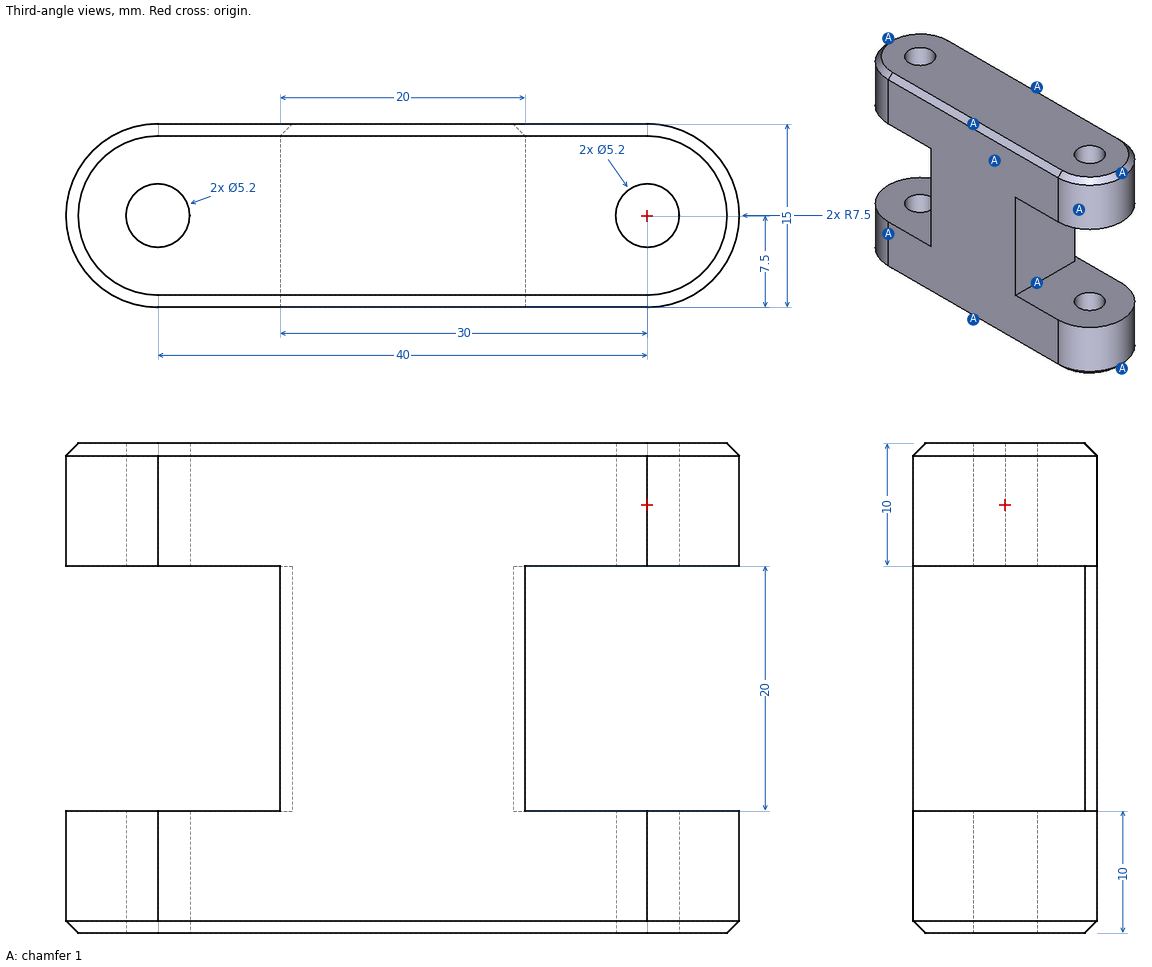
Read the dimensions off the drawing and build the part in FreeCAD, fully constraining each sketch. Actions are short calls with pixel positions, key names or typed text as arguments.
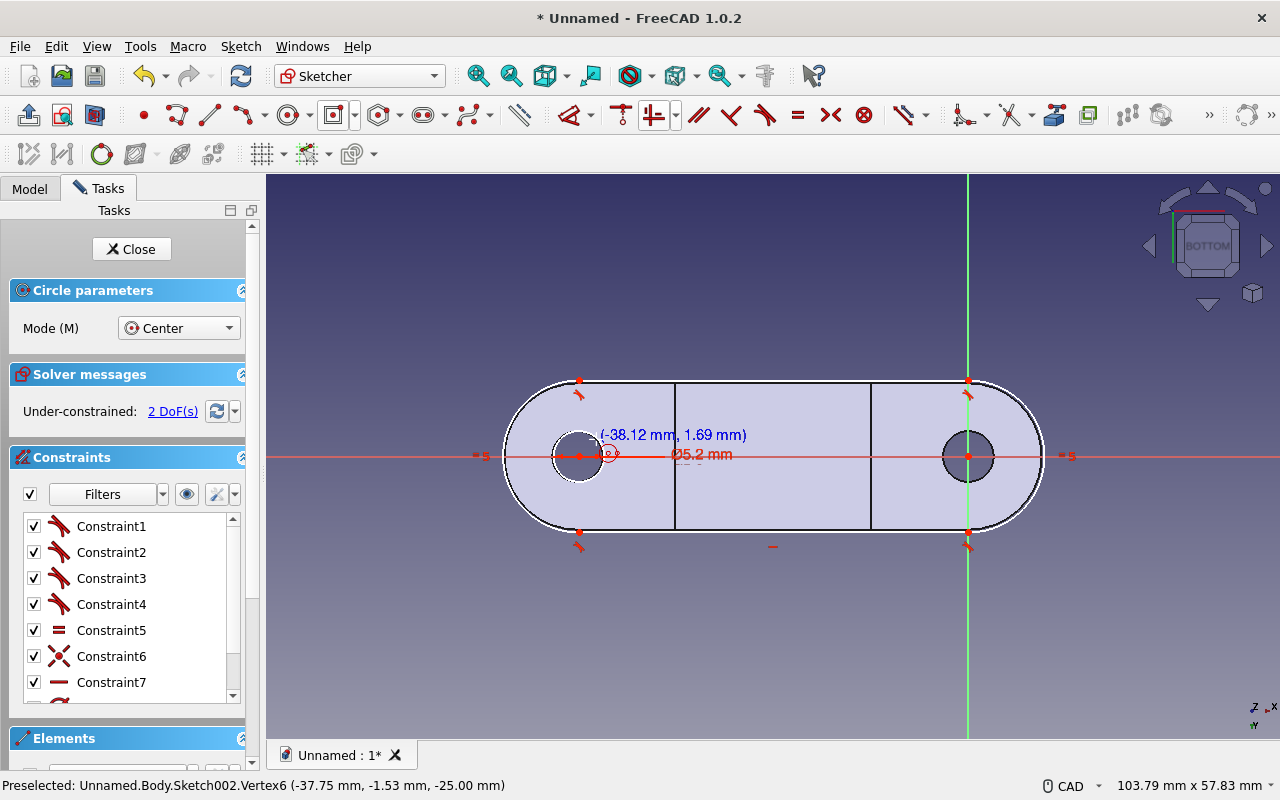
click(968, 457)
move(986, 439)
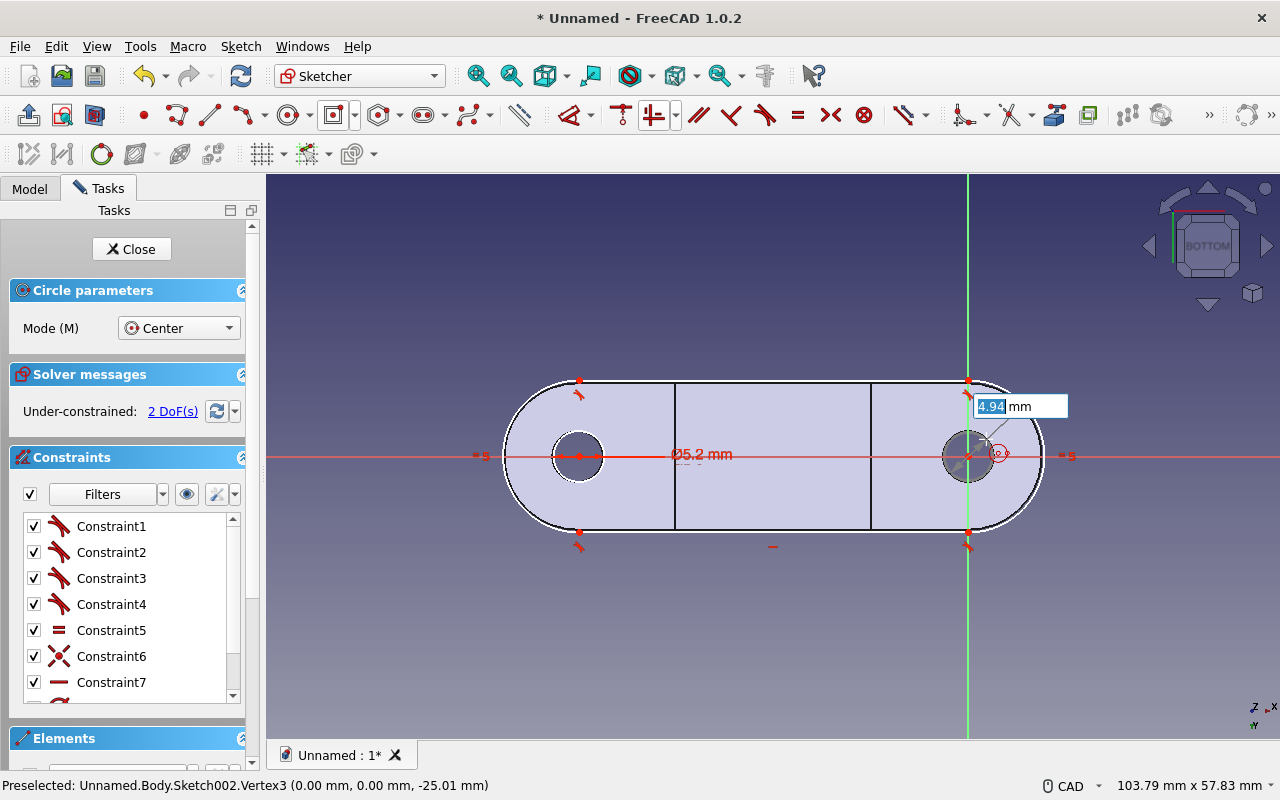
text(5.2)
key(Return)
key(Escape)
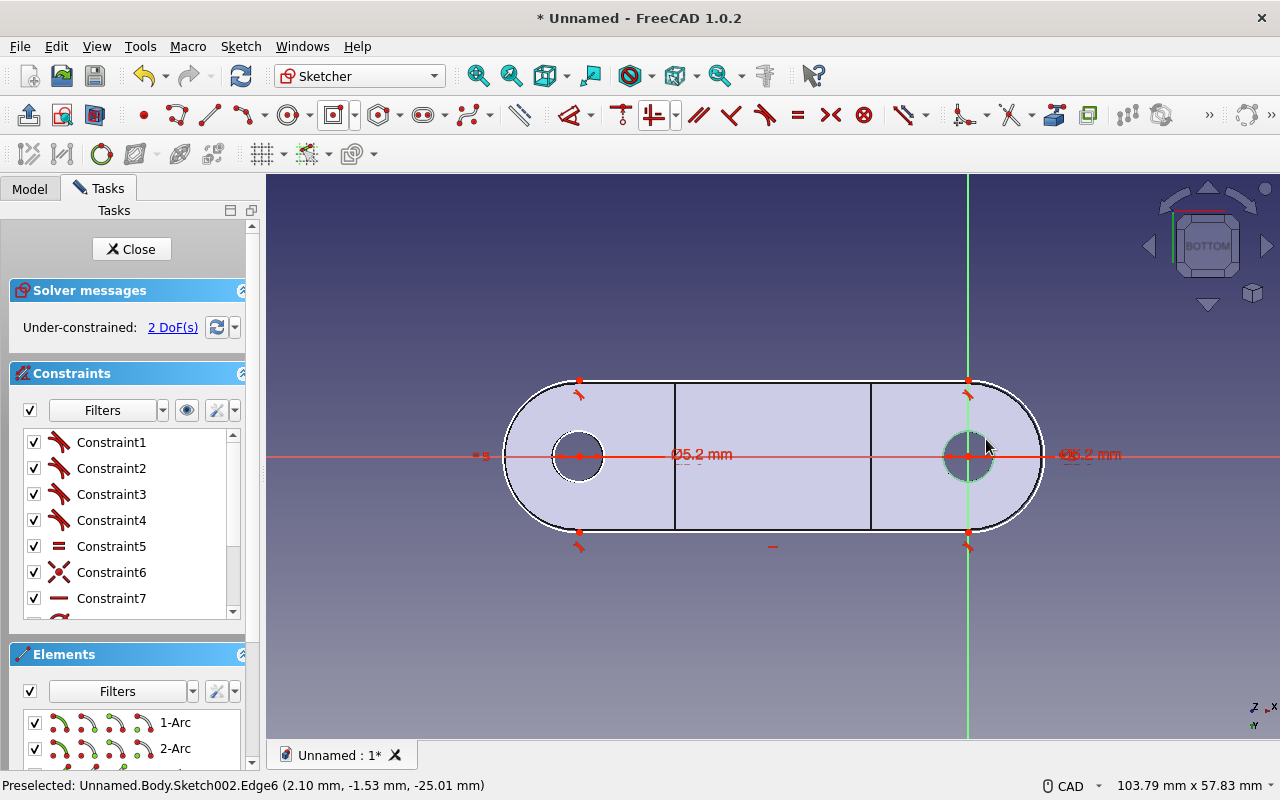
key(d)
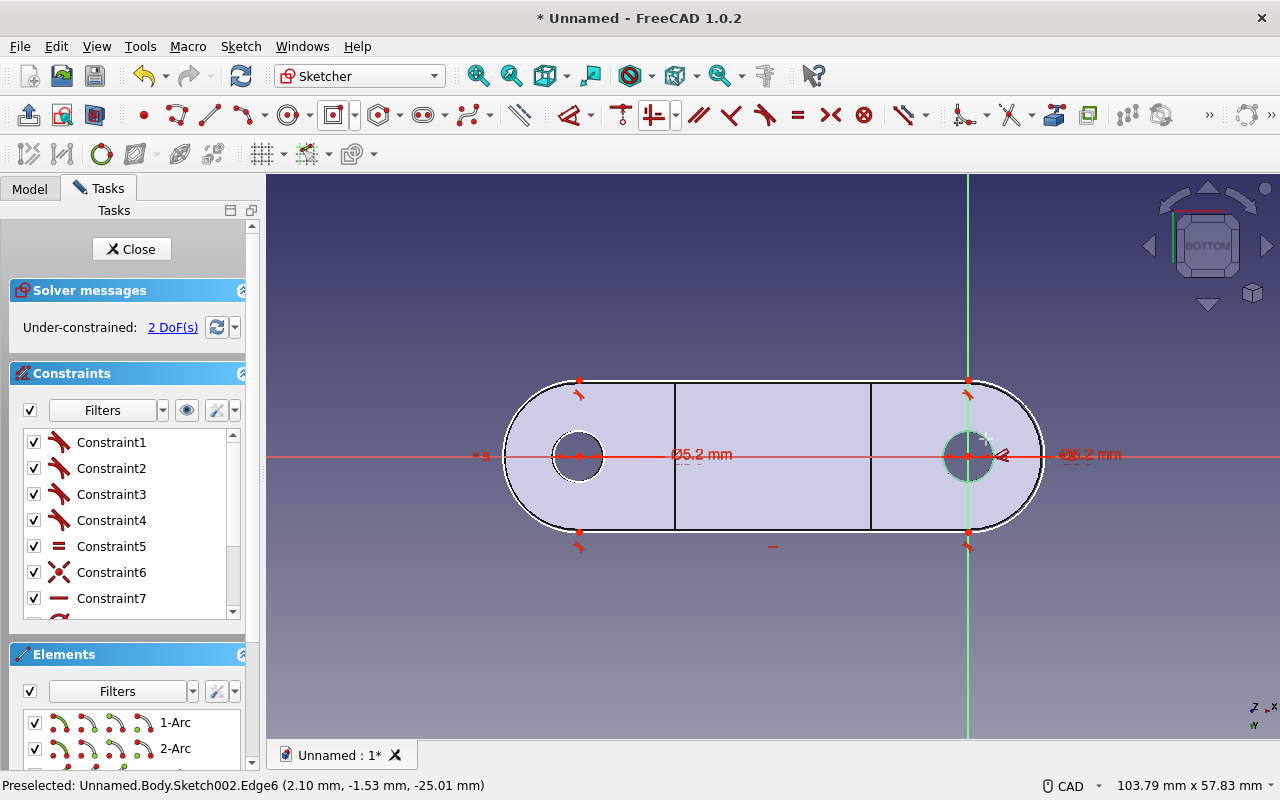
click(1030, 501)
click(1056, 520)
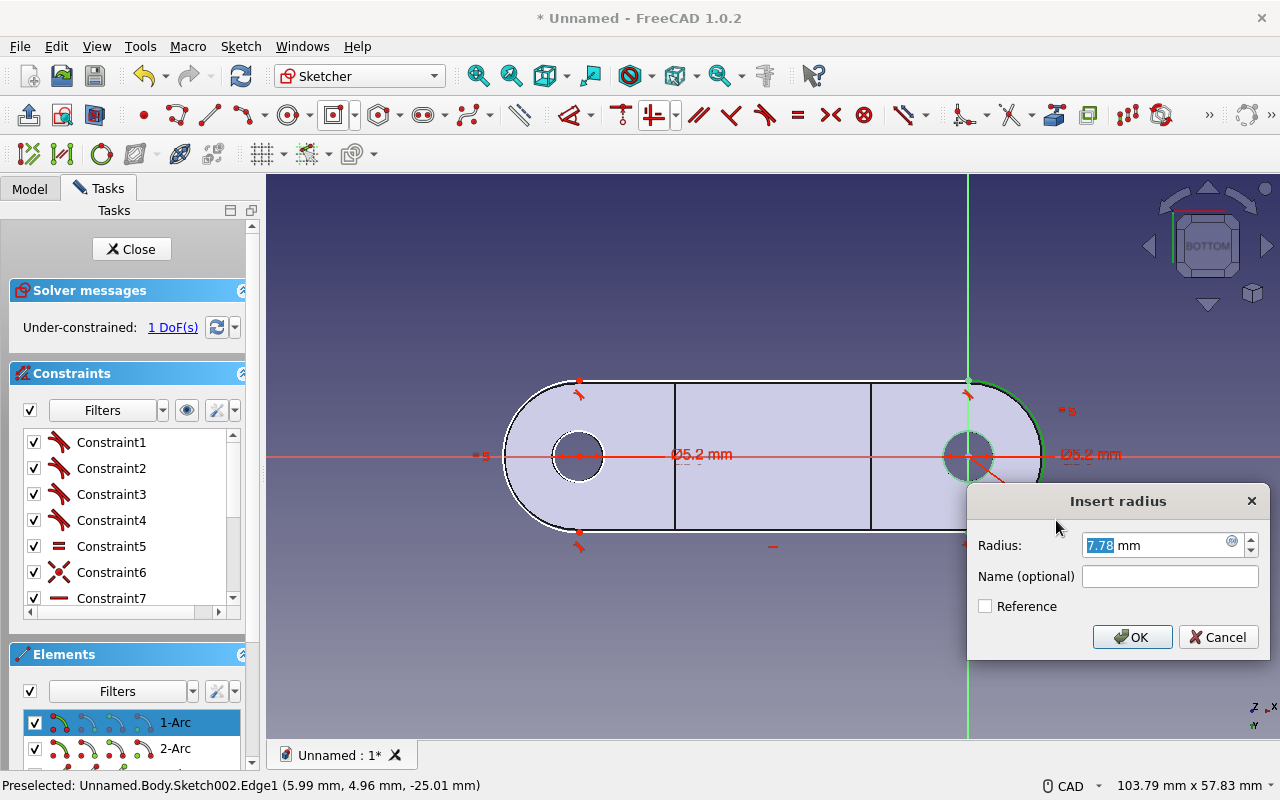
text(7.5)
key(Return)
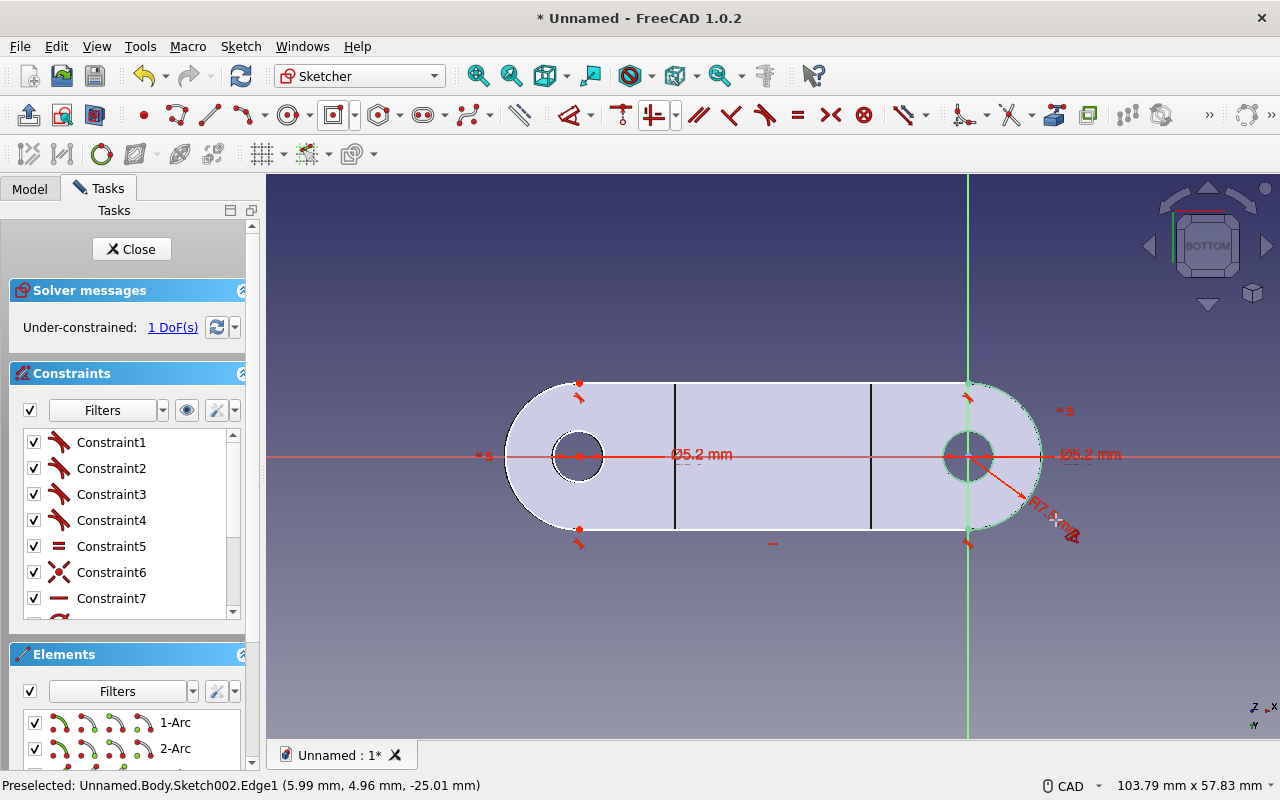
click(852, 530)
click(774, 564)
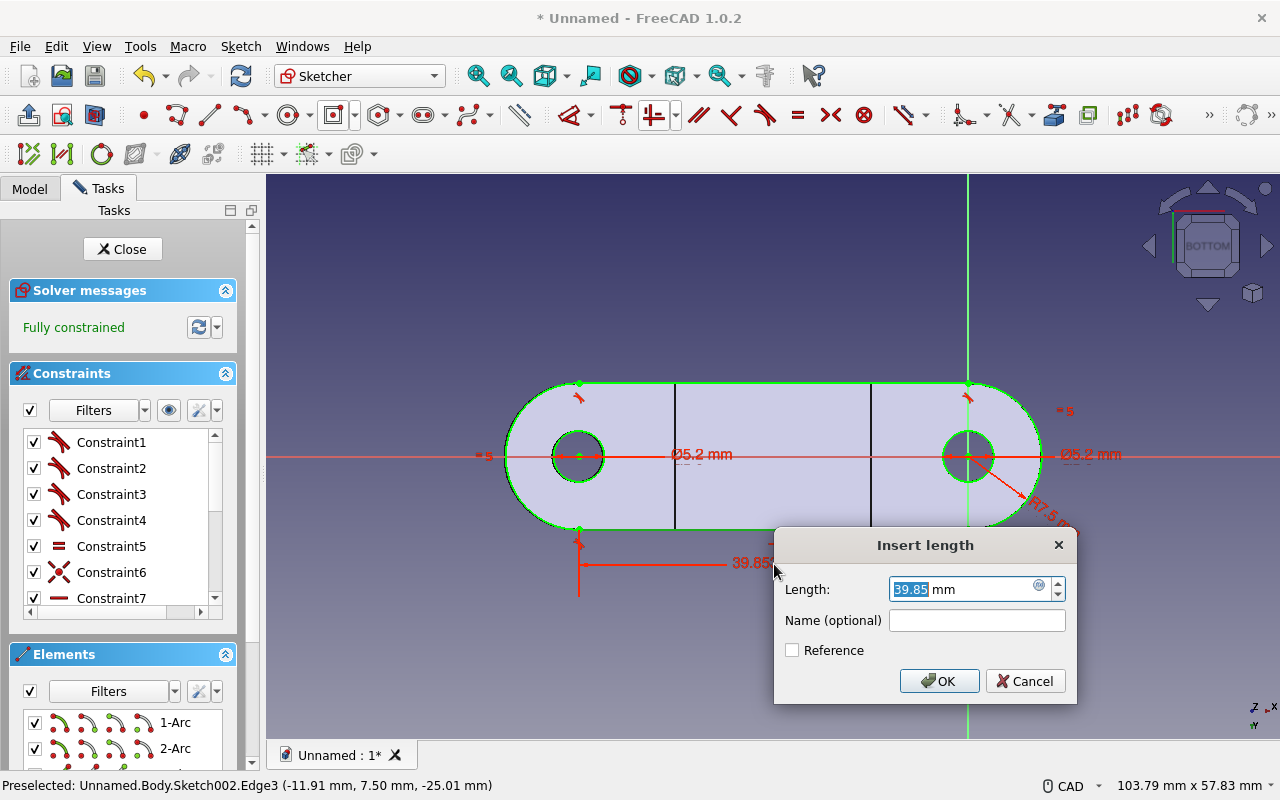
text(40)
key(Return)
key(Escape)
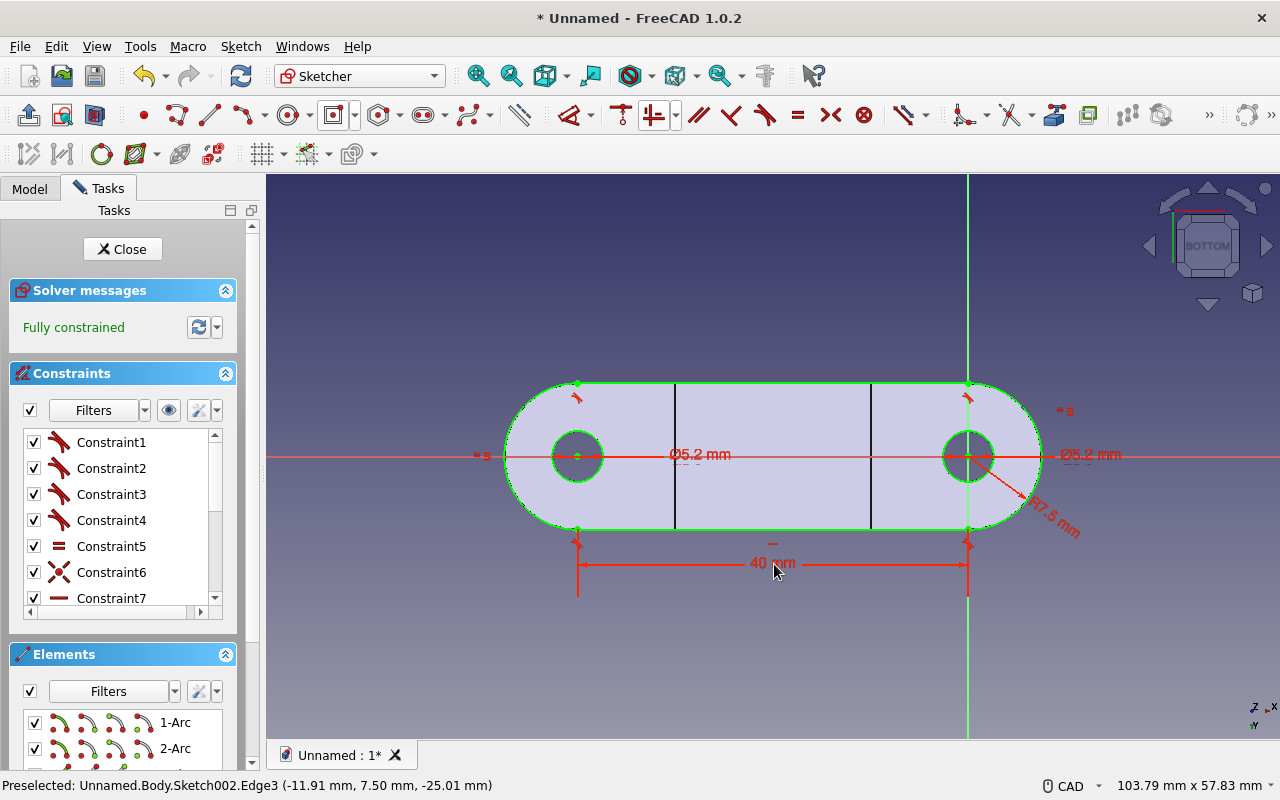
click(123, 249)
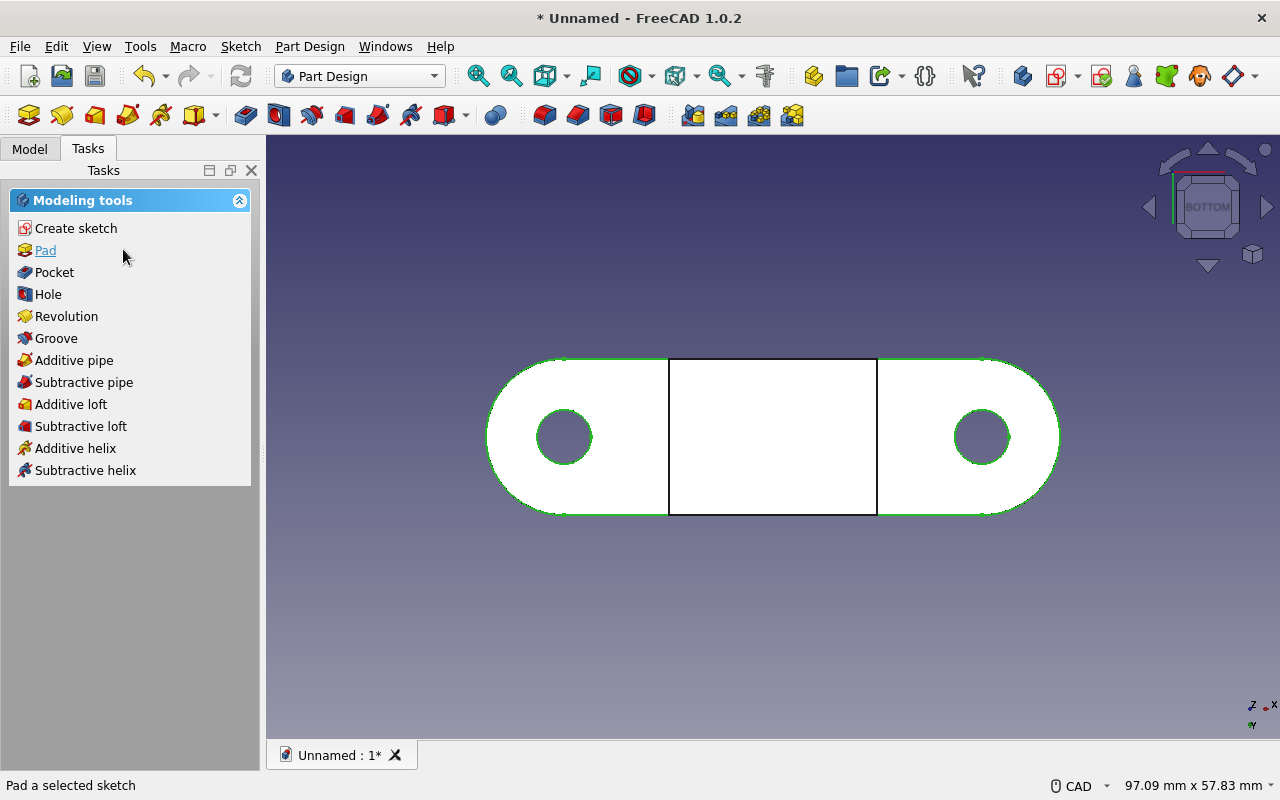
click(29, 116)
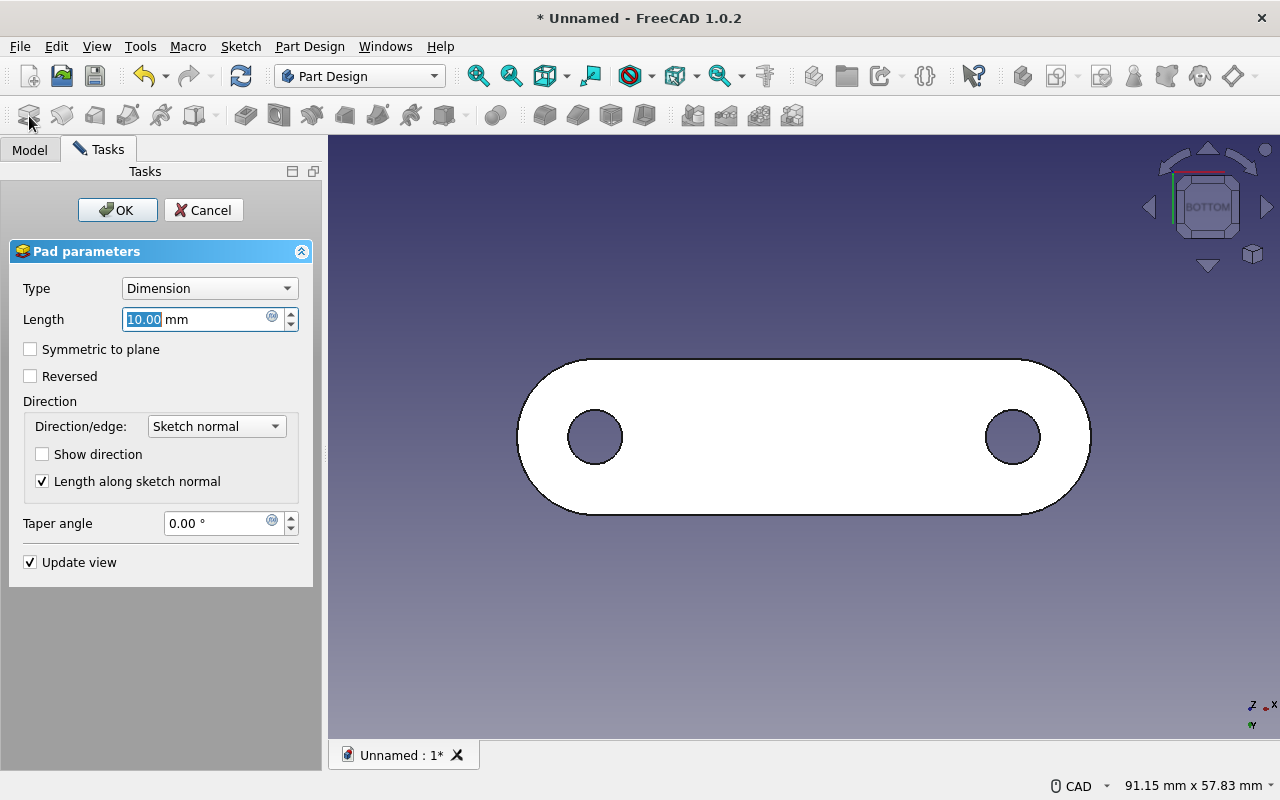
text(10)
key(Tab)